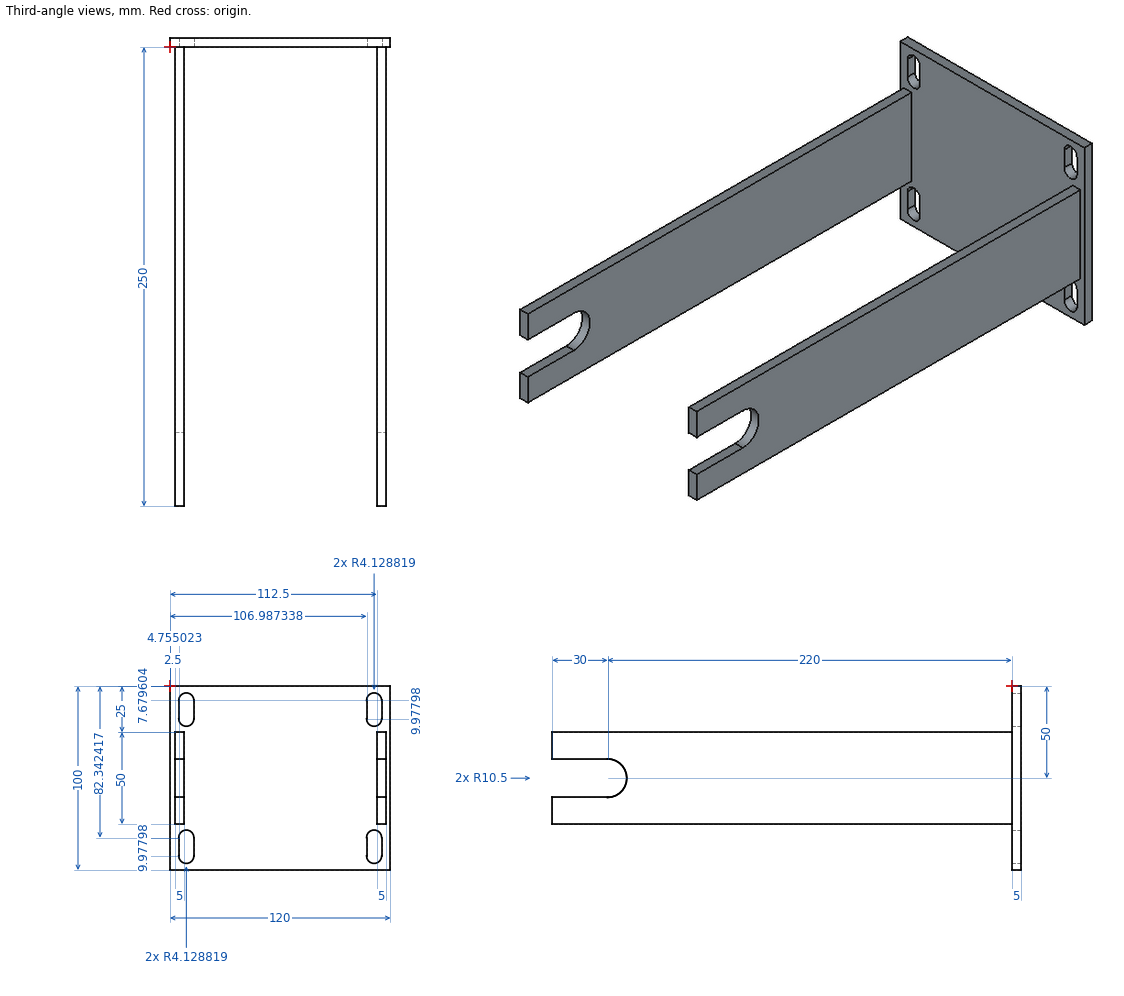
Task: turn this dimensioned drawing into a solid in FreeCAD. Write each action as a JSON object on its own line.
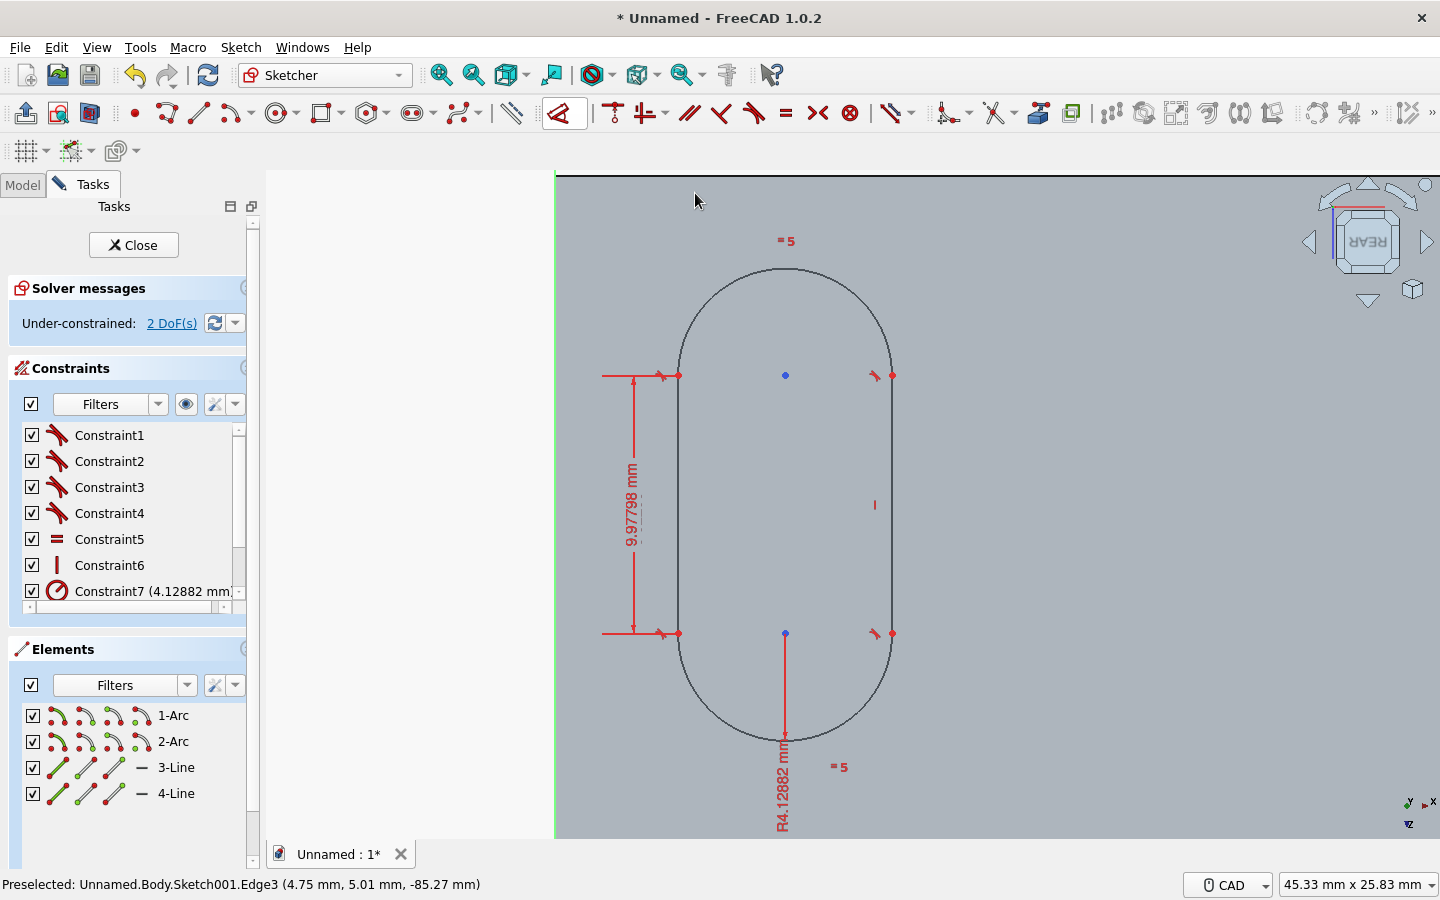
{"action": "left_click", "coordinate": [678, 634]}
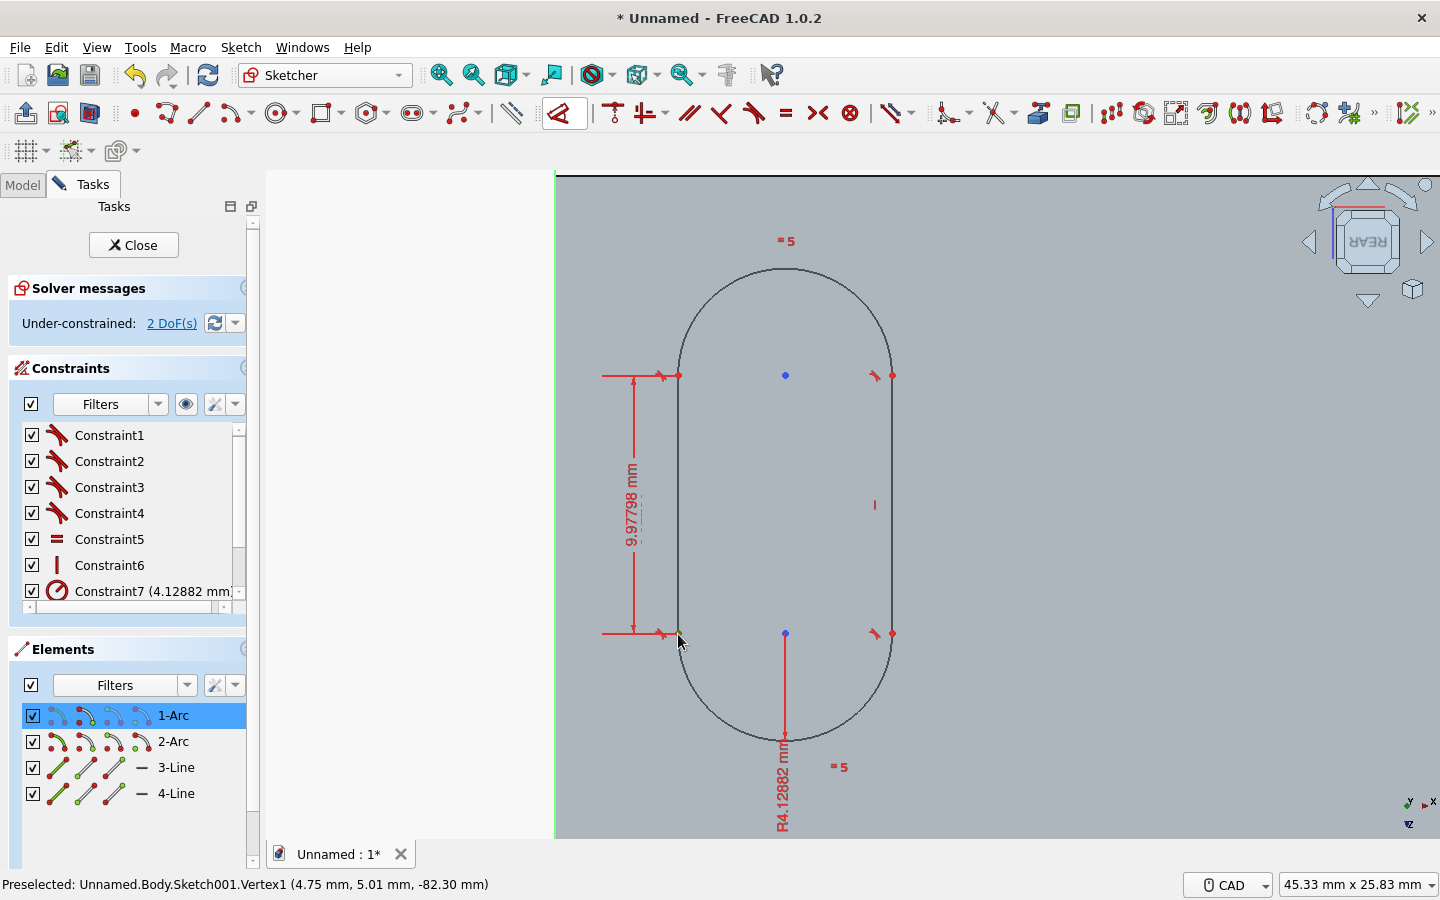
{"action": "left_click", "coordinate": [582, 114]}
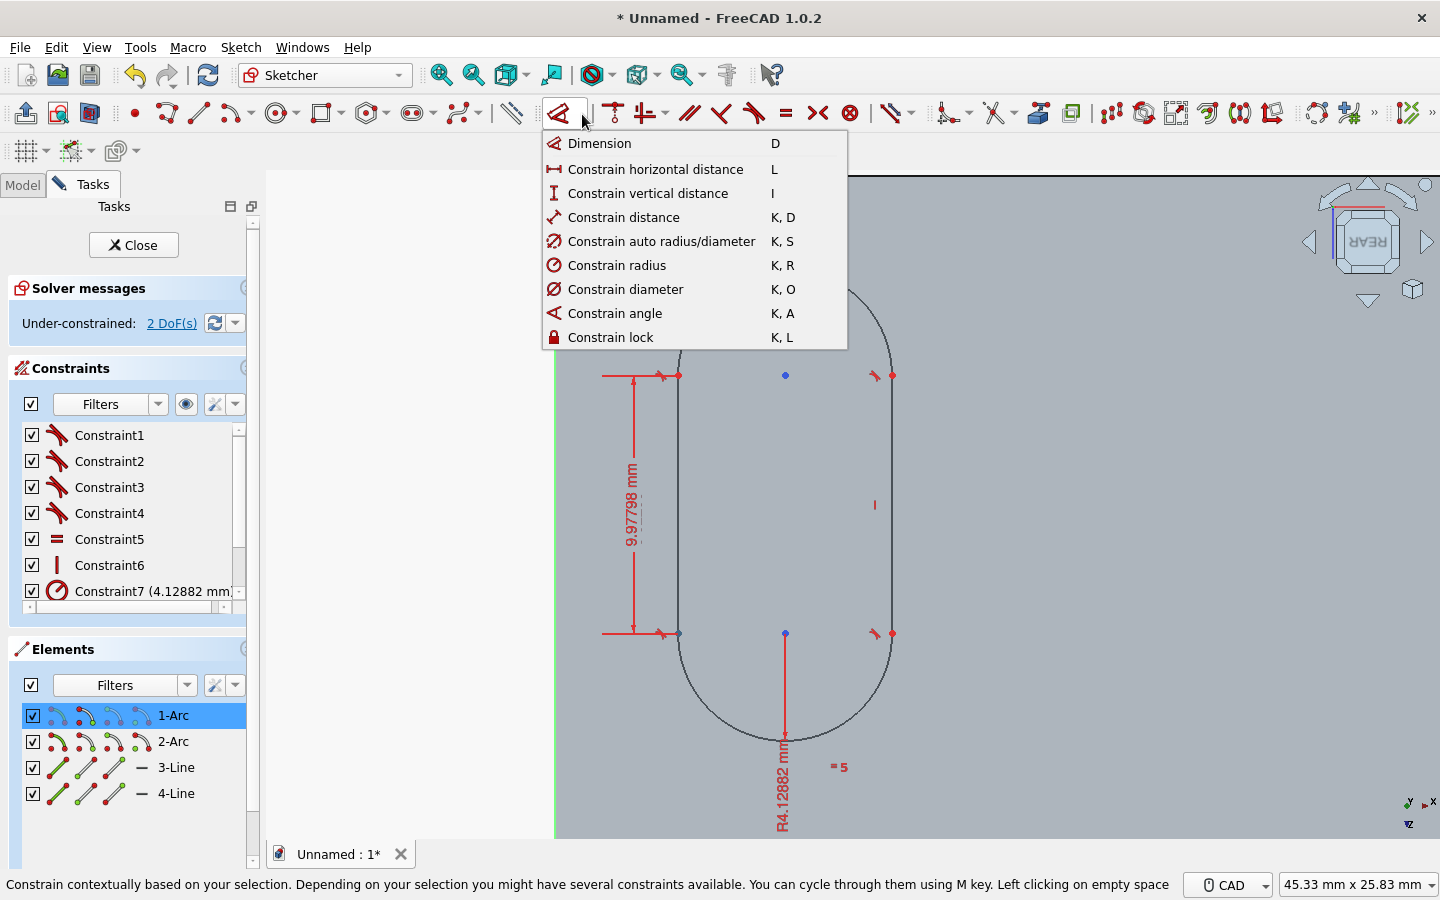
{"action": "left_click", "coordinate": [695, 169]}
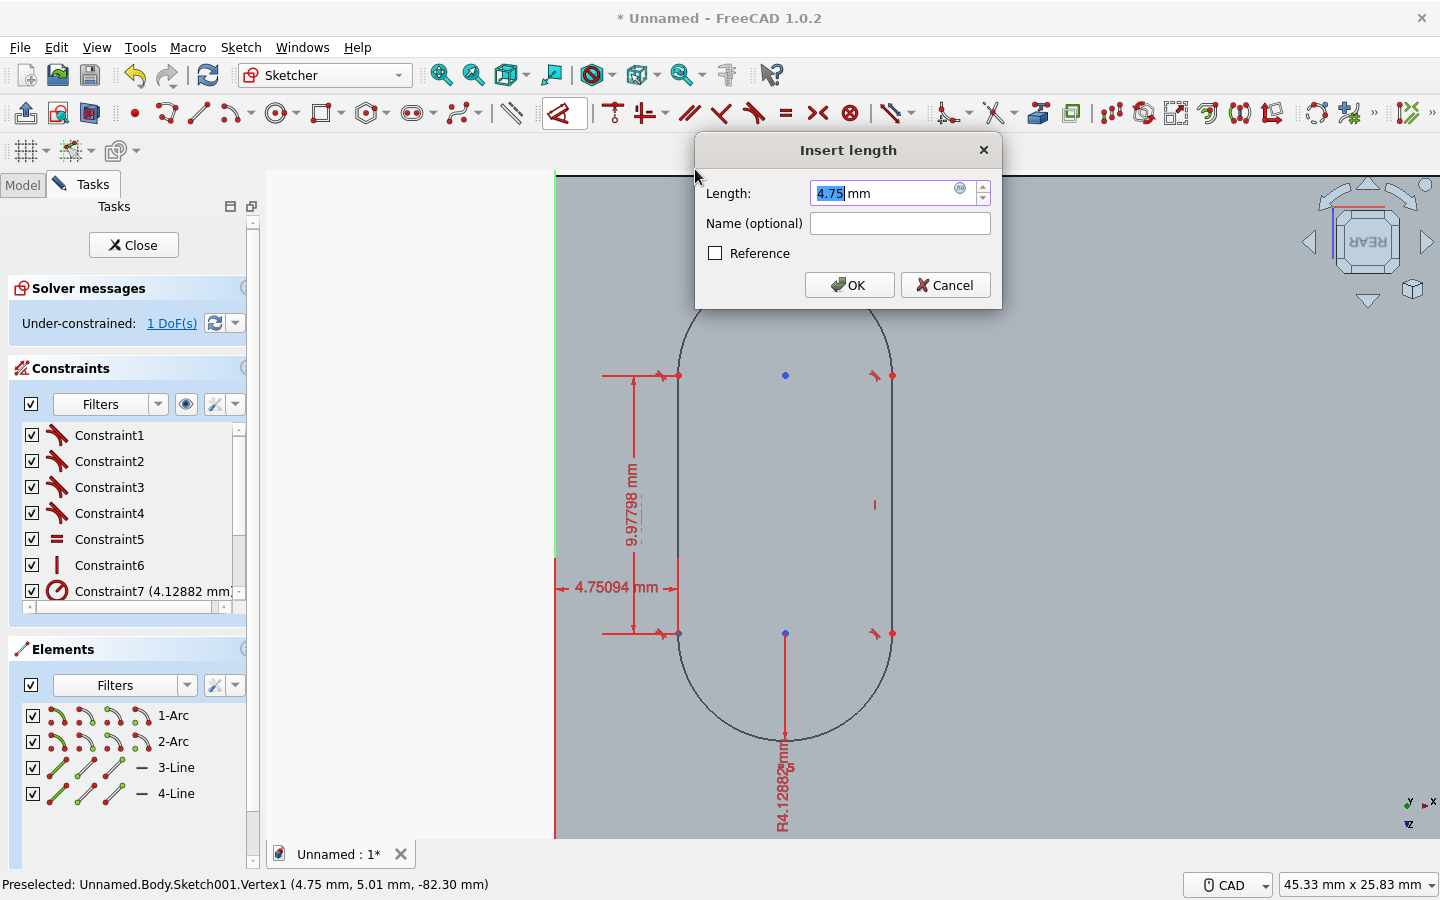
{"action": "type", "text": "4.755023"}
{"action": "key", "text": "Return"}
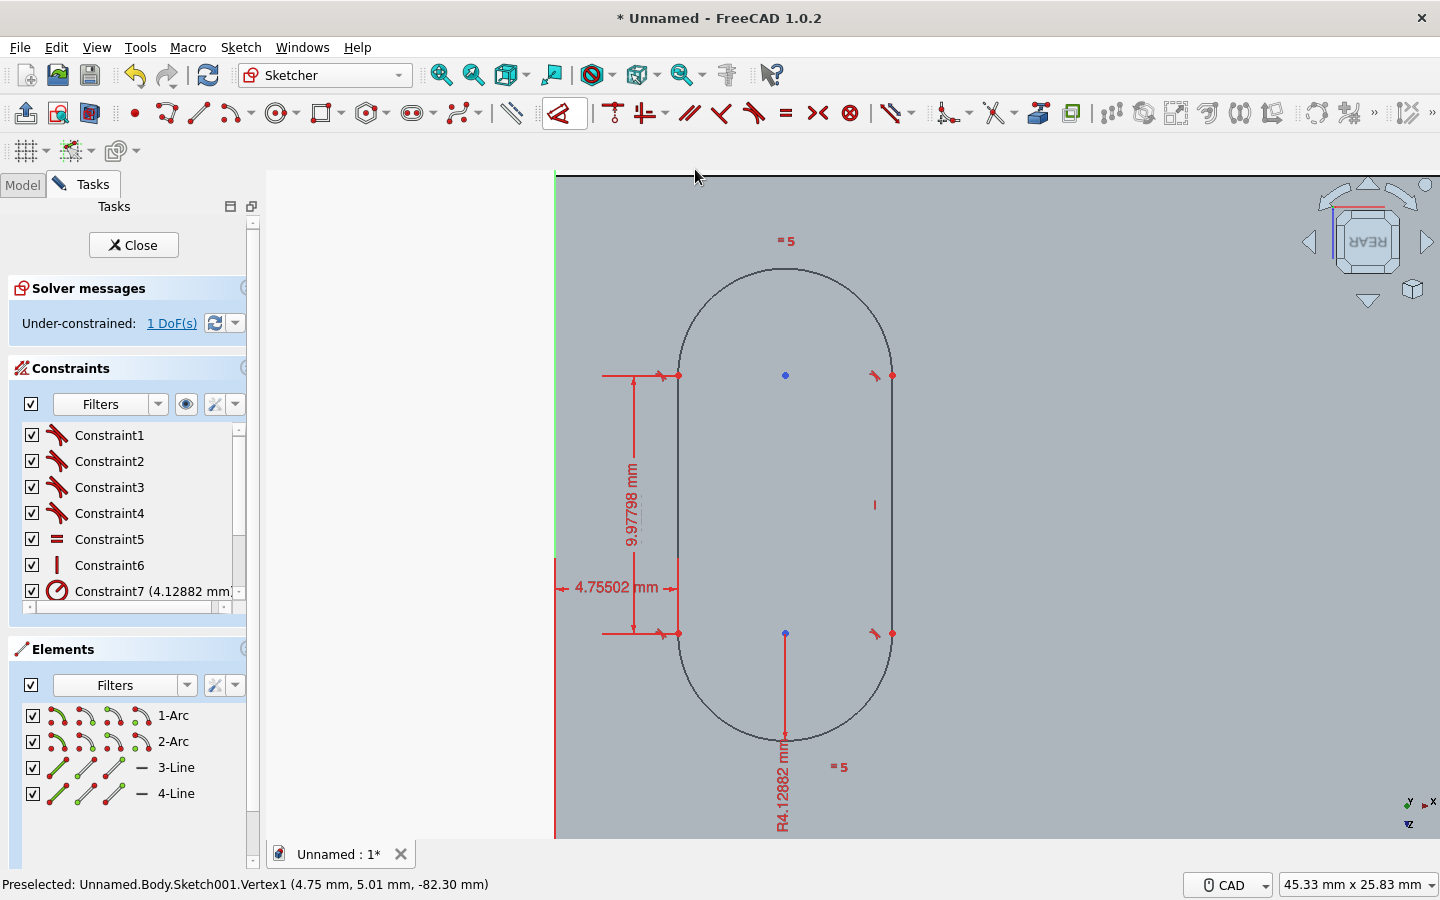
{"action": "left_click", "coordinate": [678, 634]}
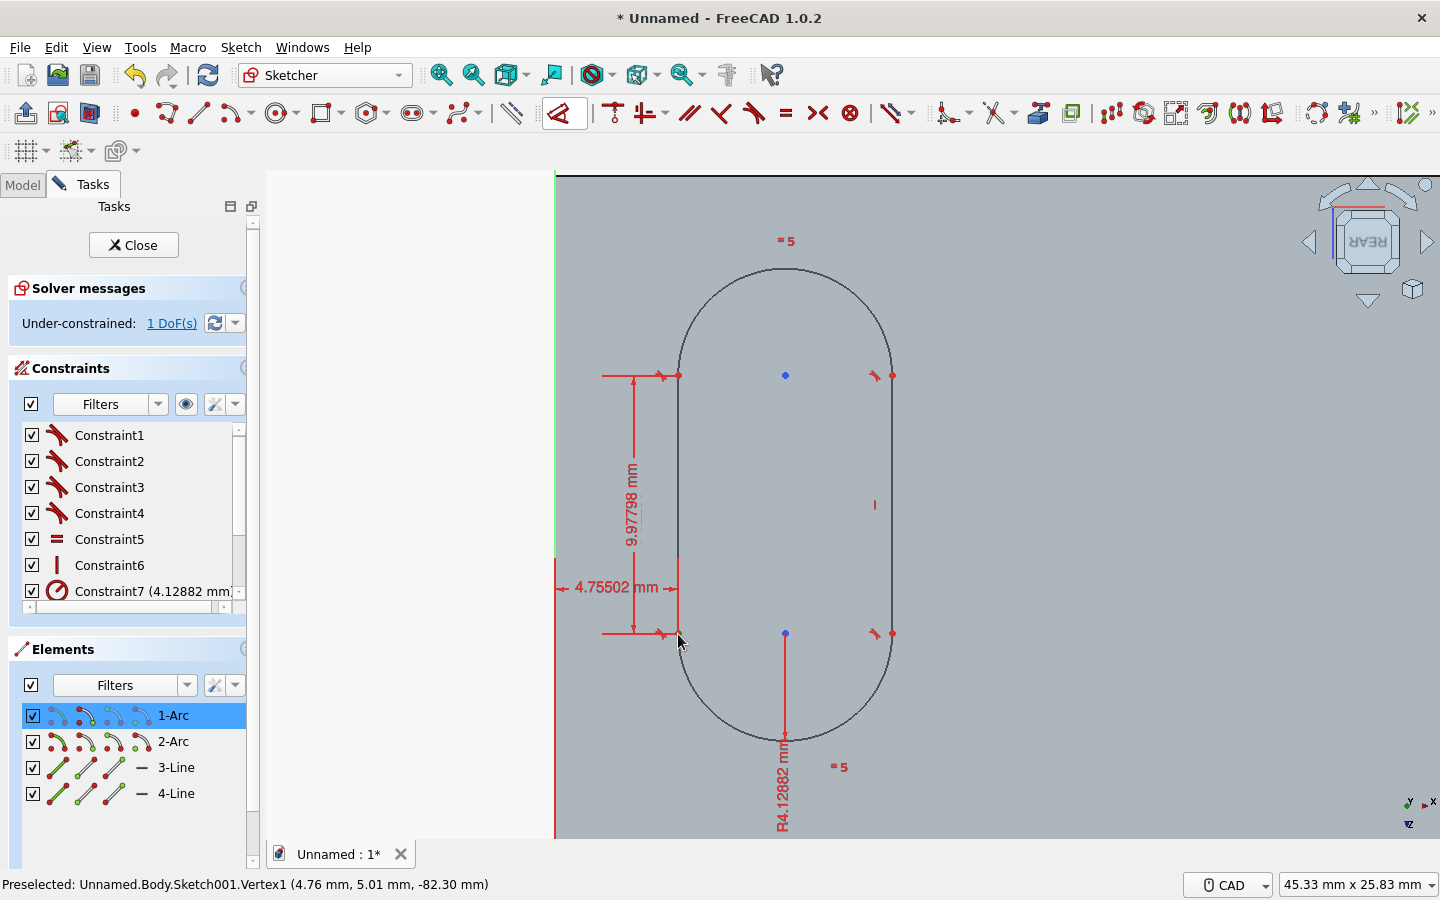
{"action": "key", "text": "i"}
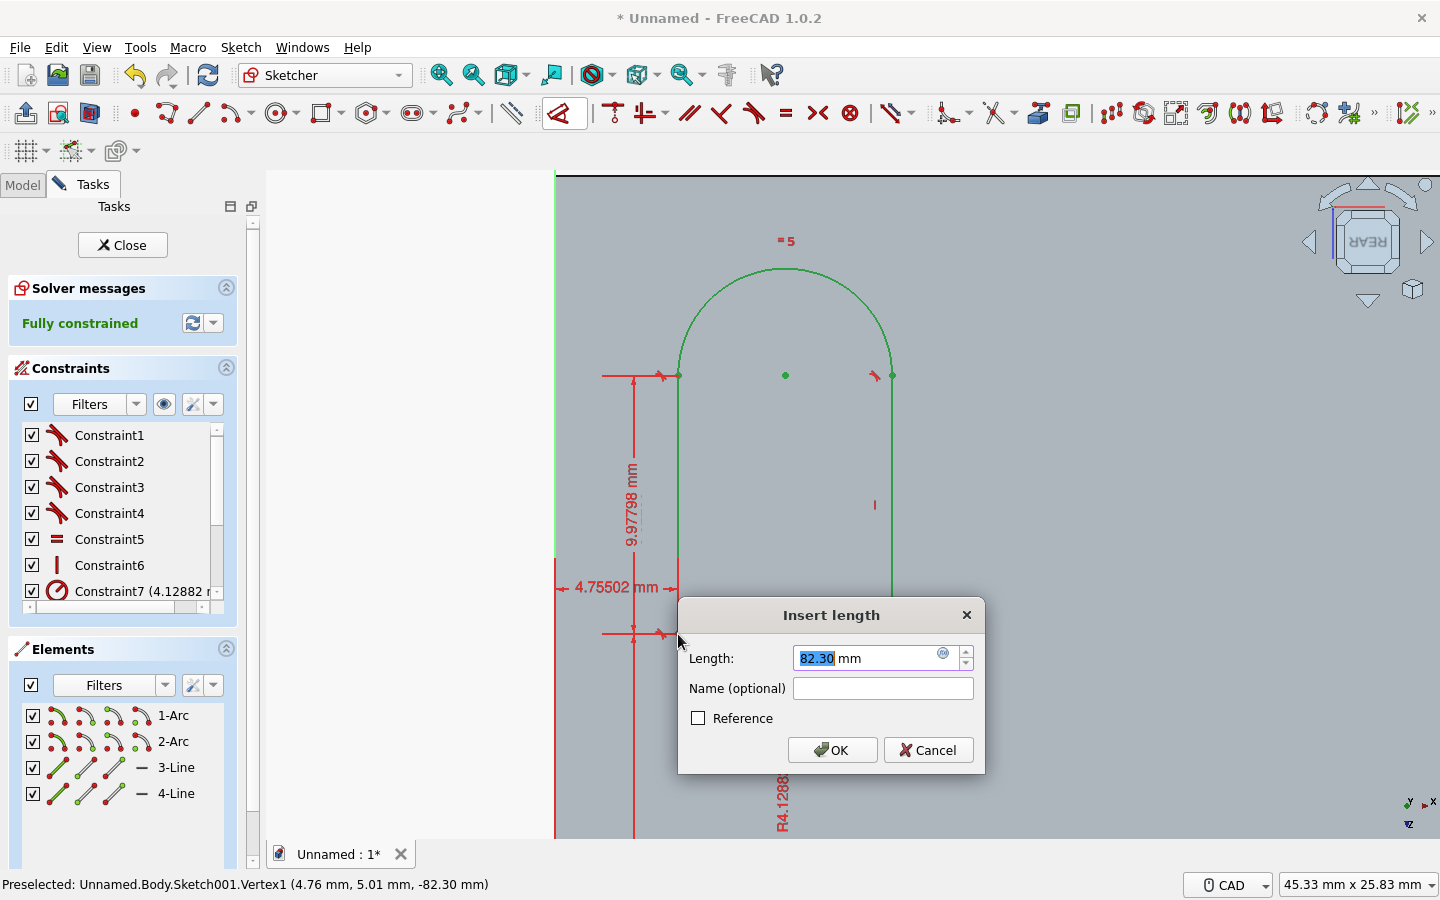
{"action": "type", "text": "82.342417"}
{"action": "key", "text": "Return"}